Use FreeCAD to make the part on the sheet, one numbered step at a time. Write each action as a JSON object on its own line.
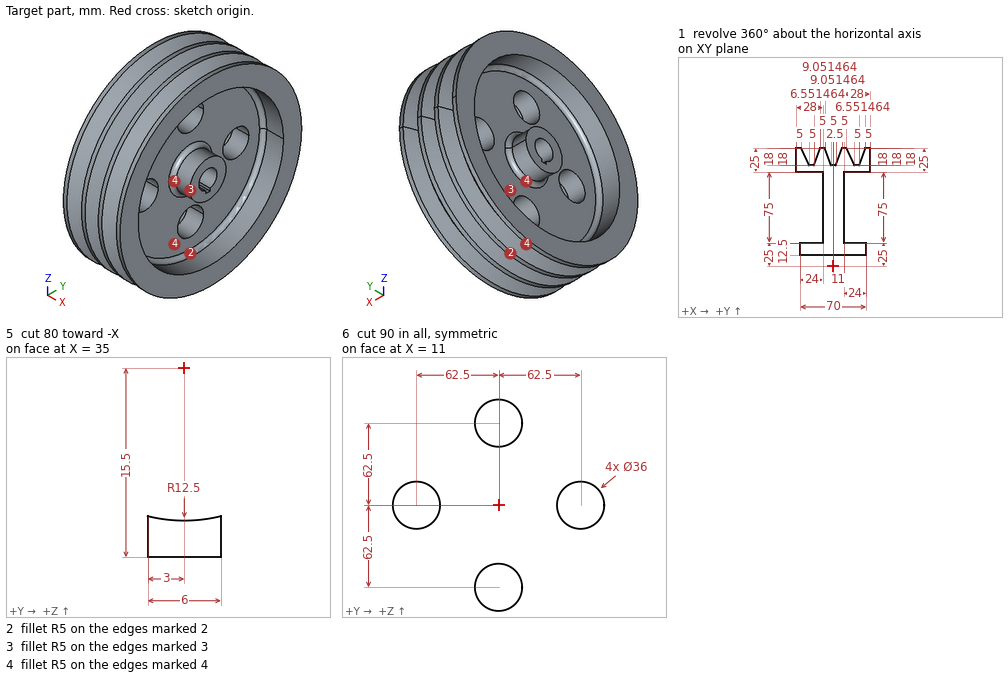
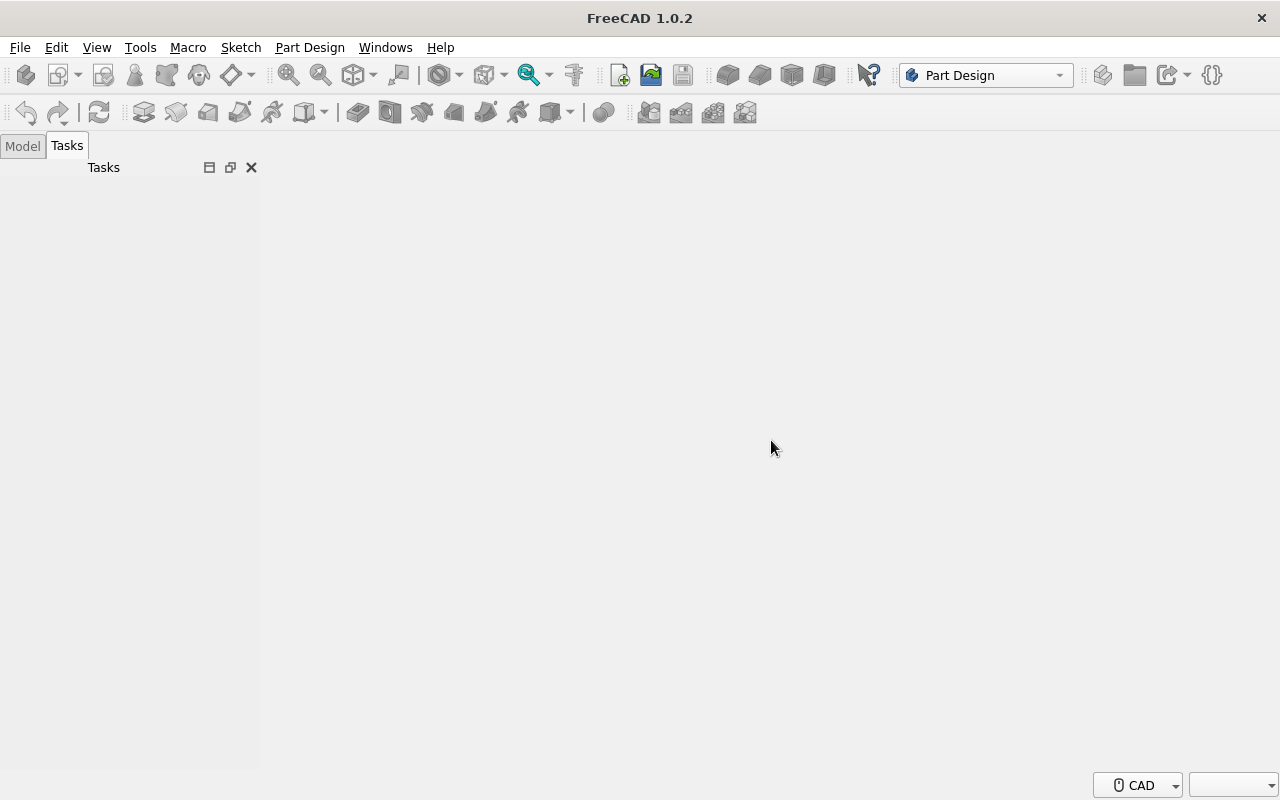
{"action": "left_click", "coordinate": [620, 76]}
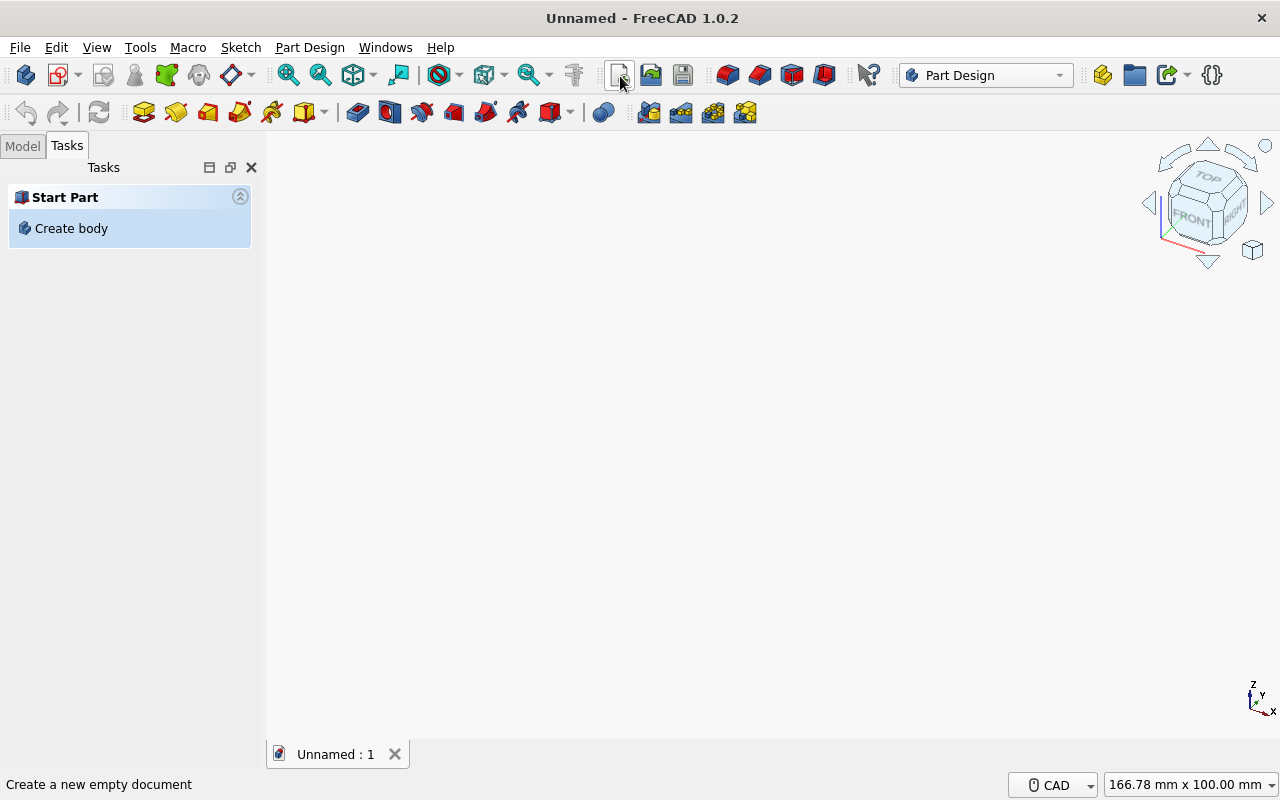
{"action": "left_click", "coordinate": [58, 76]}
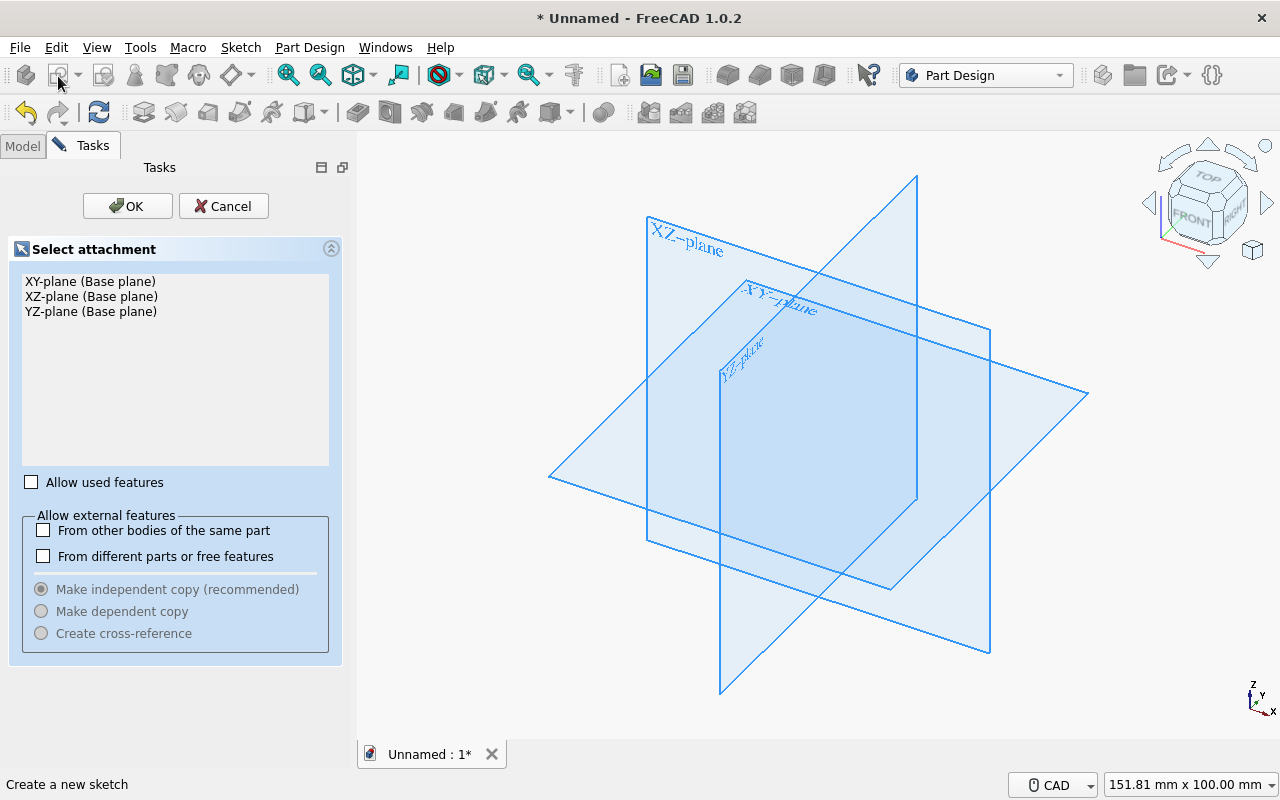
{"action": "left_click", "coordinate": [82, 282]}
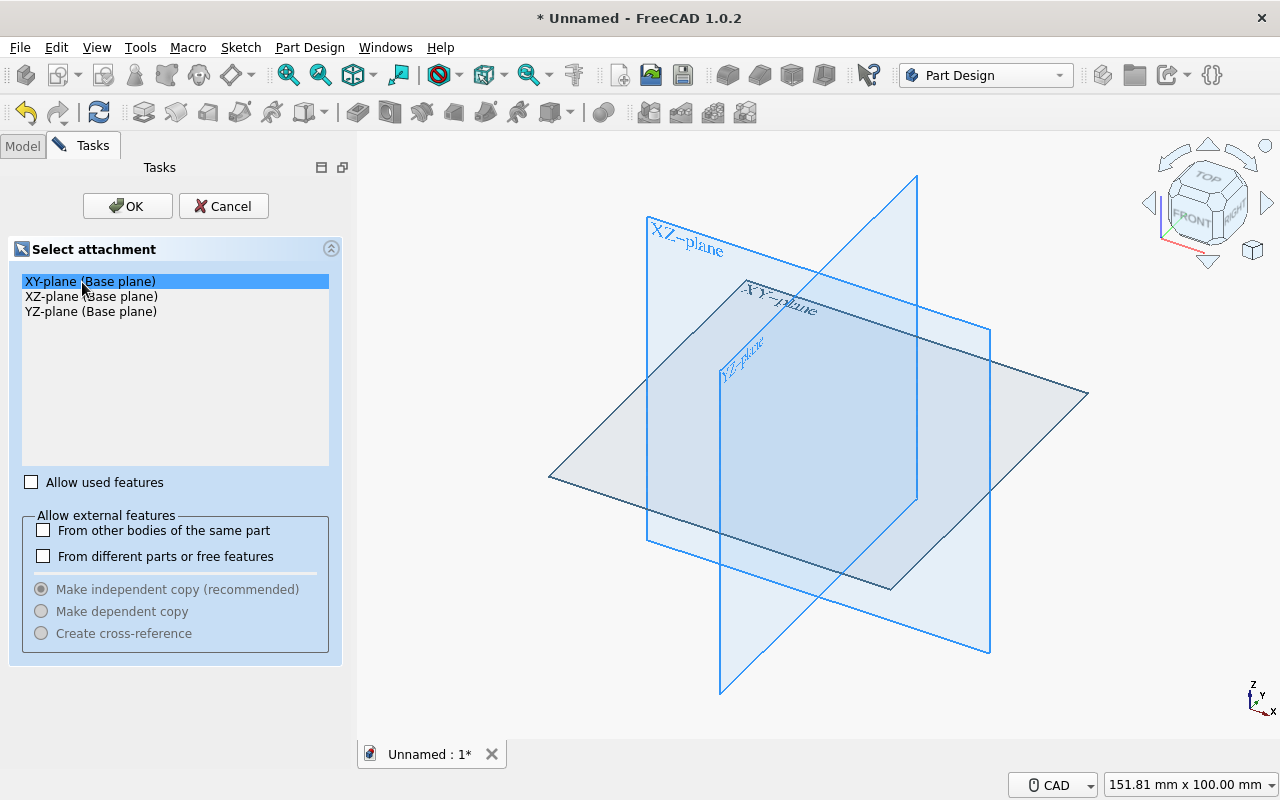
{"action": "left_click", "coordinate": [128, 206]}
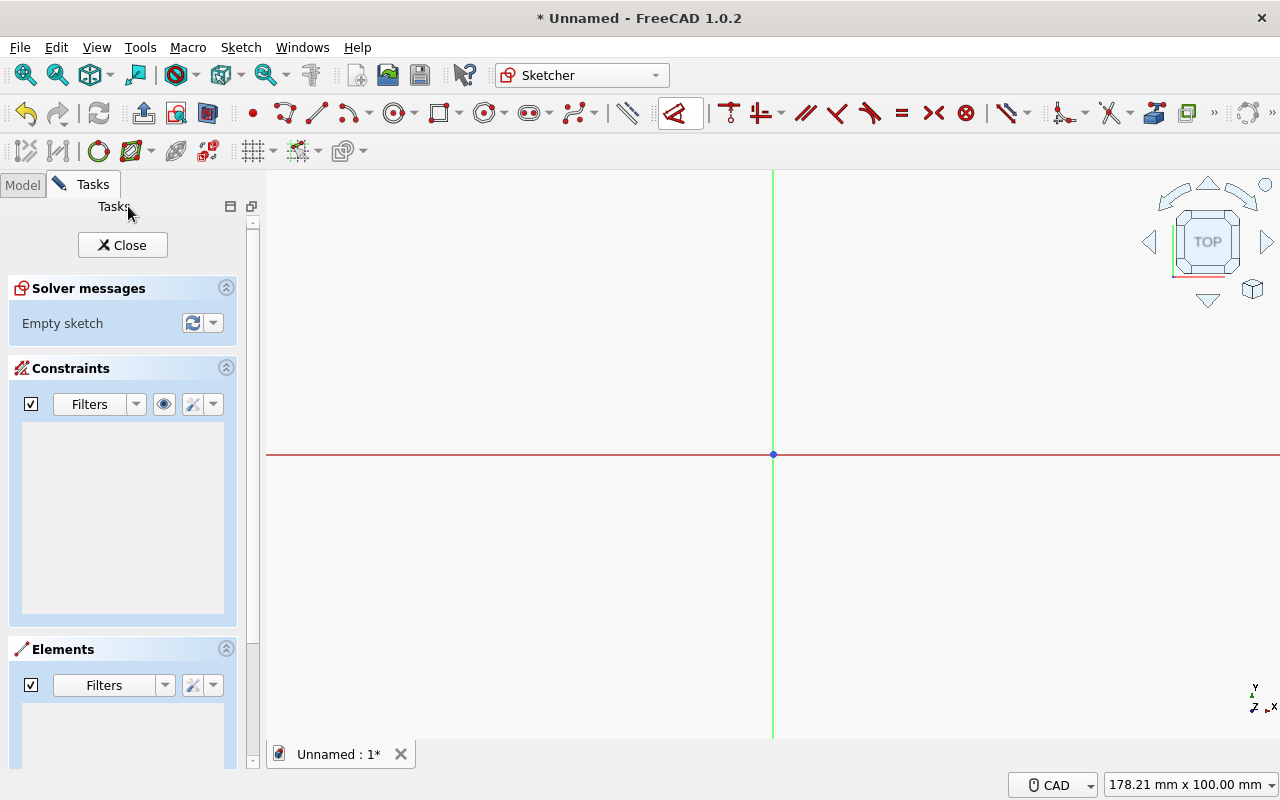
{"action": "scroll", "coordinate": [649, 711], "scroll_direction": "down", "scroll_amount": 4}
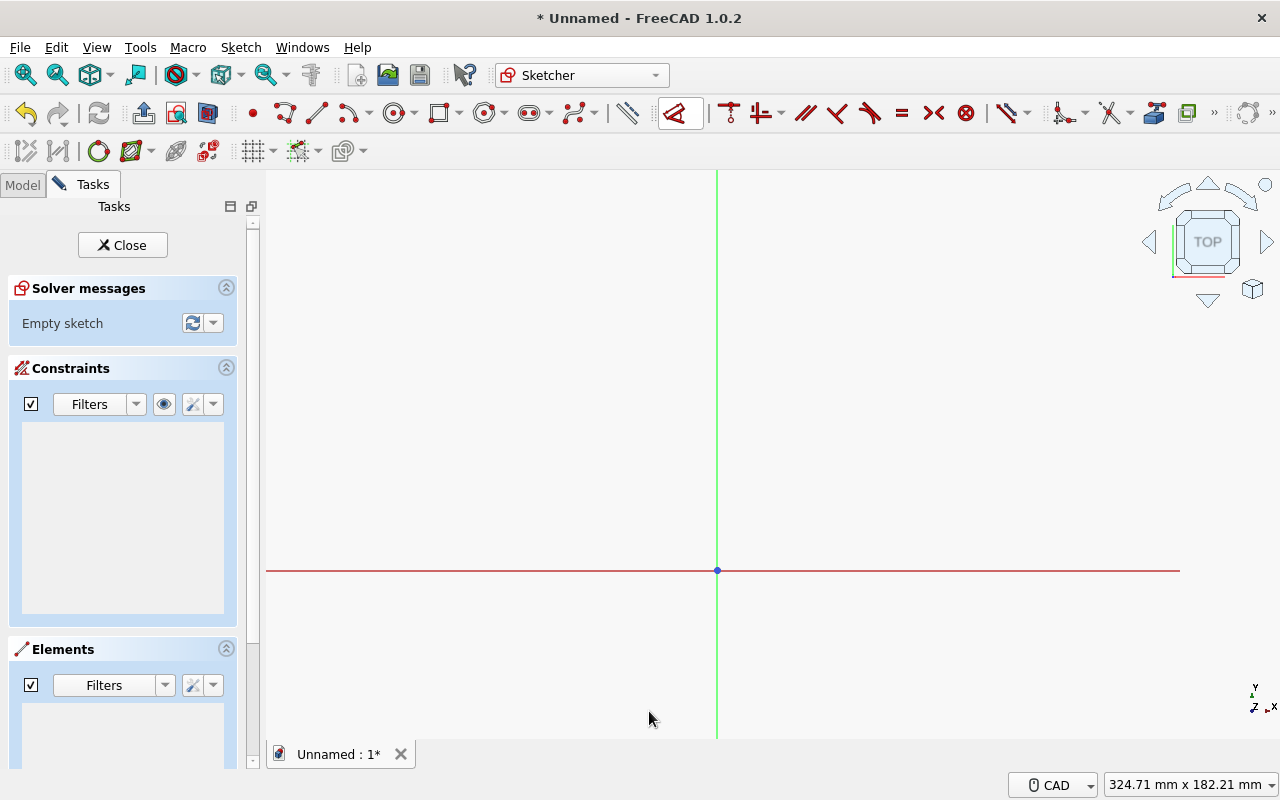
{"action": "left_click", "coordinate": [286, 114]}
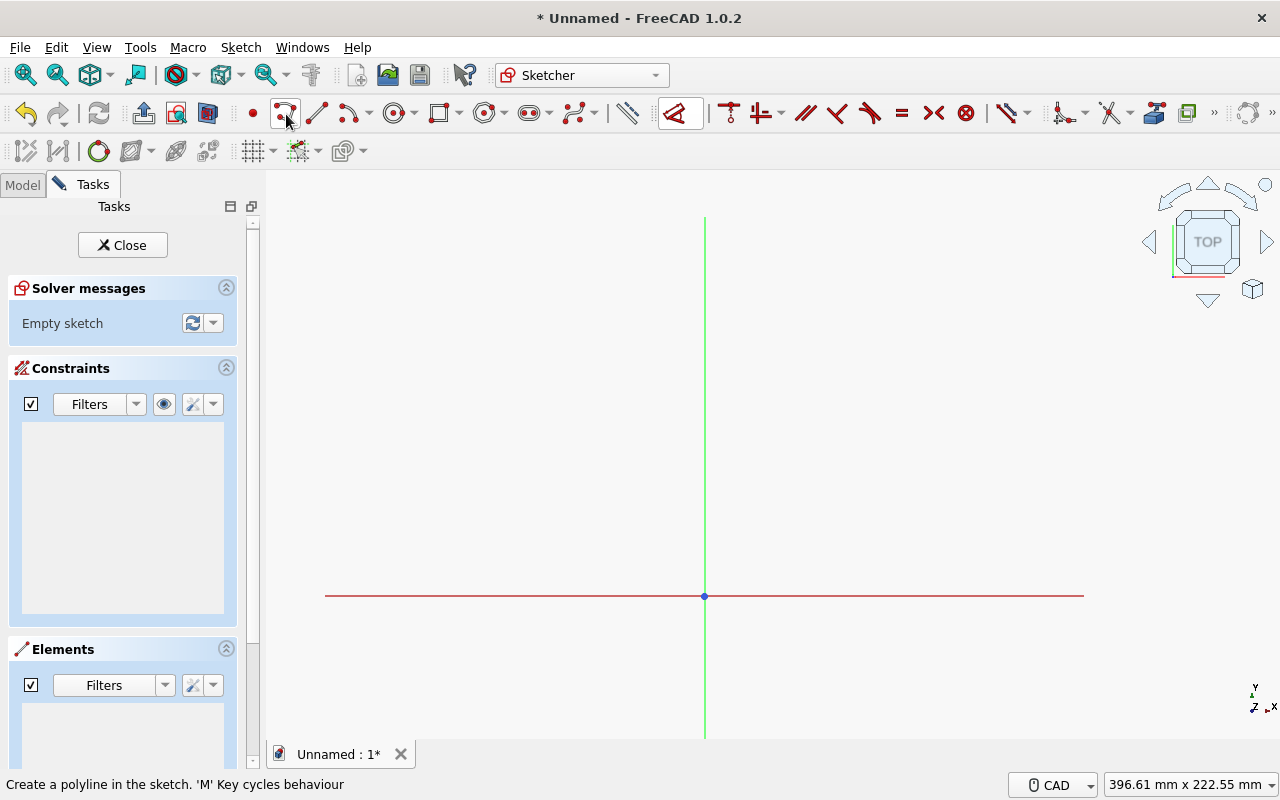
{"action": "left_click", "coordinate": [733, 532]}
{"action": "left_click", "coordinate": [733, 341]}
{"action": "left_click", "coordinate": [805, 341]}
{"action": "left_click", "coordinate": [805, 277]}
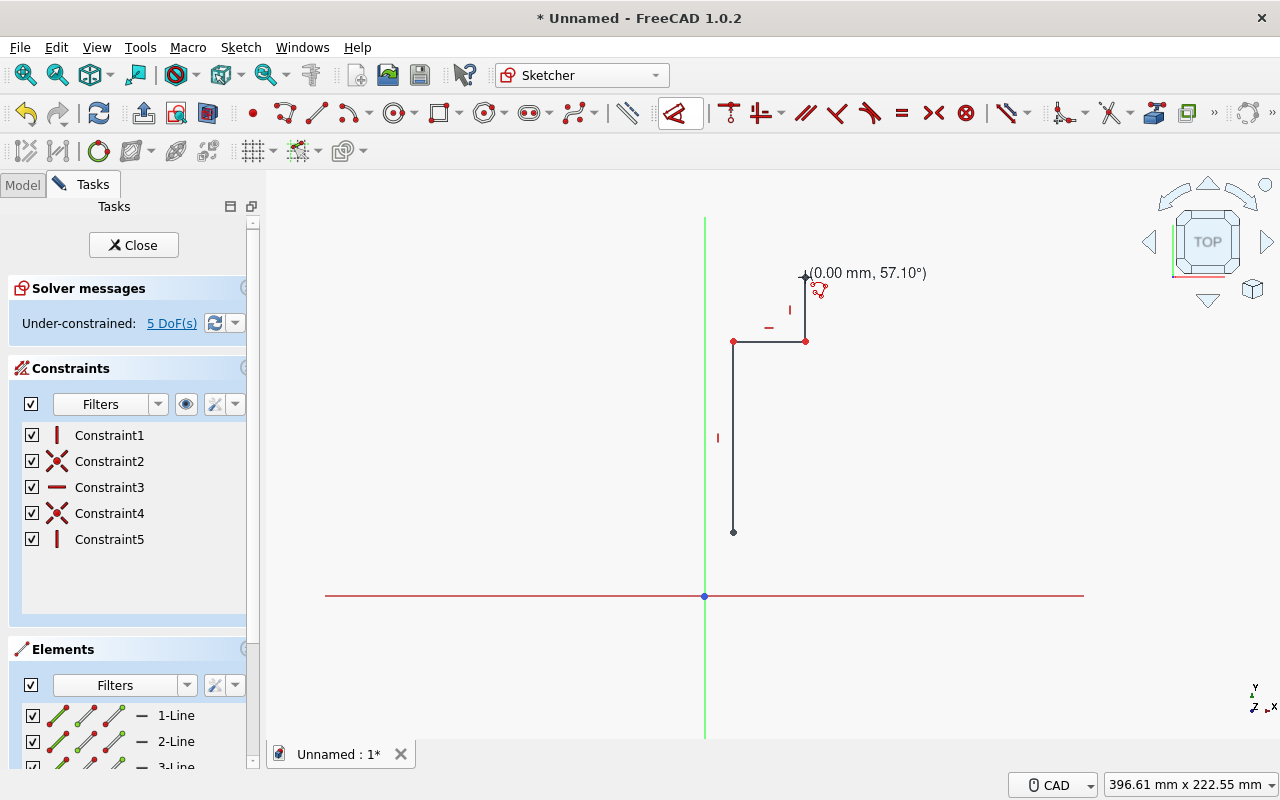
{"action": "scroll", "coordinate": [792, 277], "scroll_direction": "up", "scroll_amount": 2}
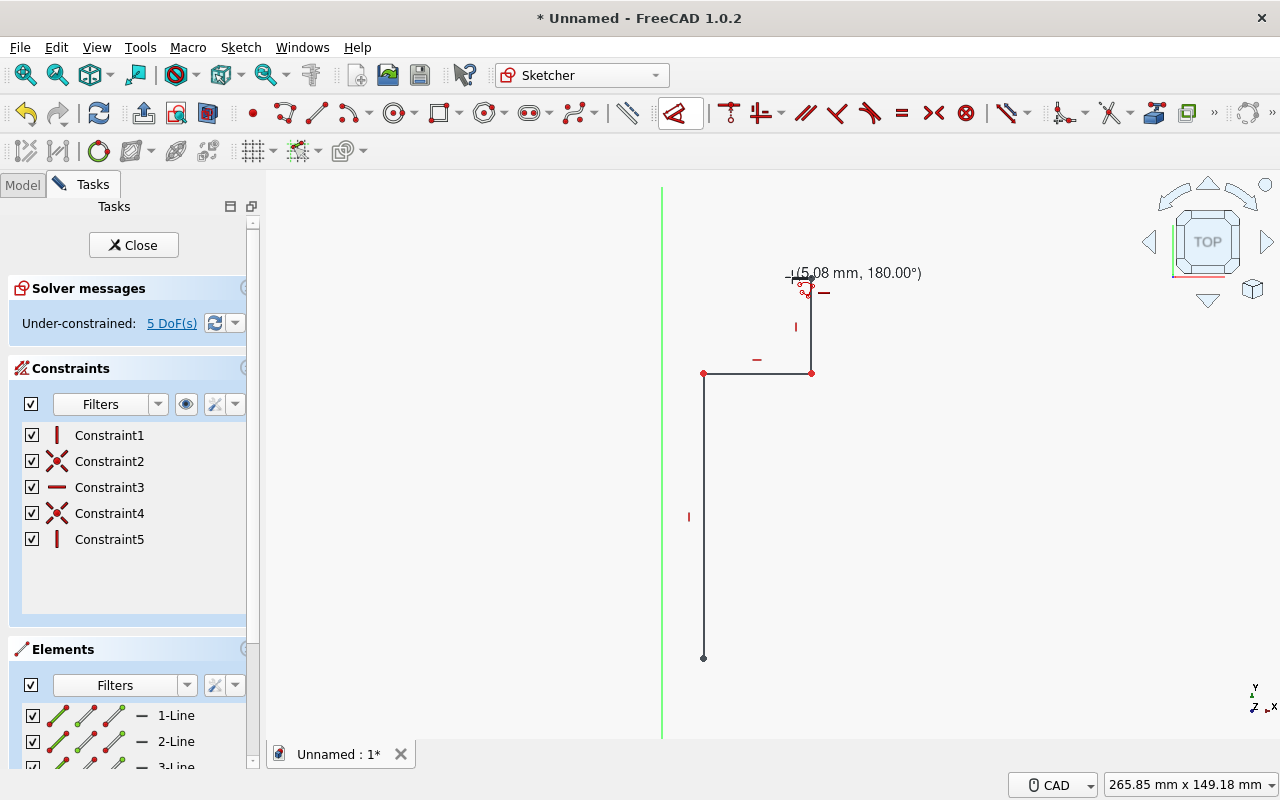
{"action": "left_click", "coordinate": [792, 277]}
{"action": "left_click", "coordinate": [767, 345]}
{"action": "left_click", "coordinate": [747, 345]}
{"action": "left_click", "coordinate": [715, 276]}
{"action": "left_click", "coordinate": [696, 276]}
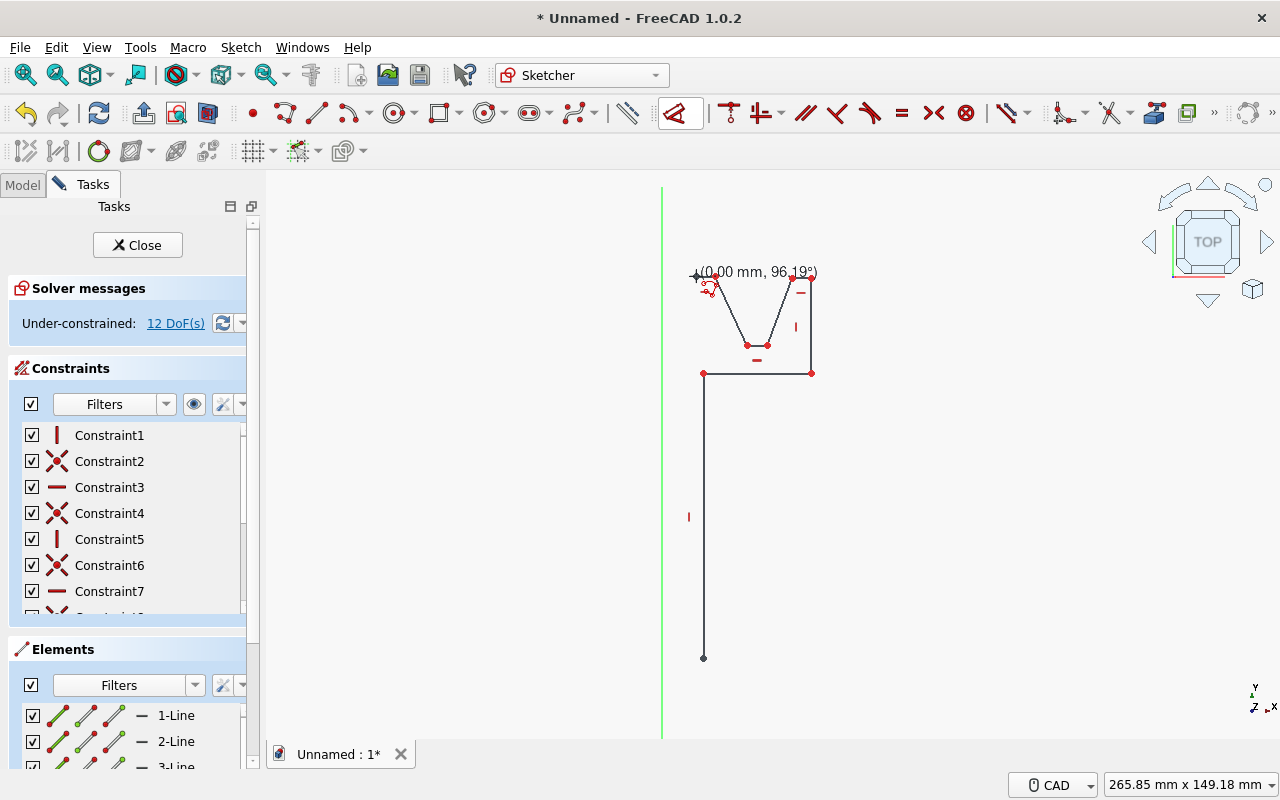
{"action": "scroll", "coordinate": [671, 345], "scroll_direction": "up", "scroll_amount": 3}